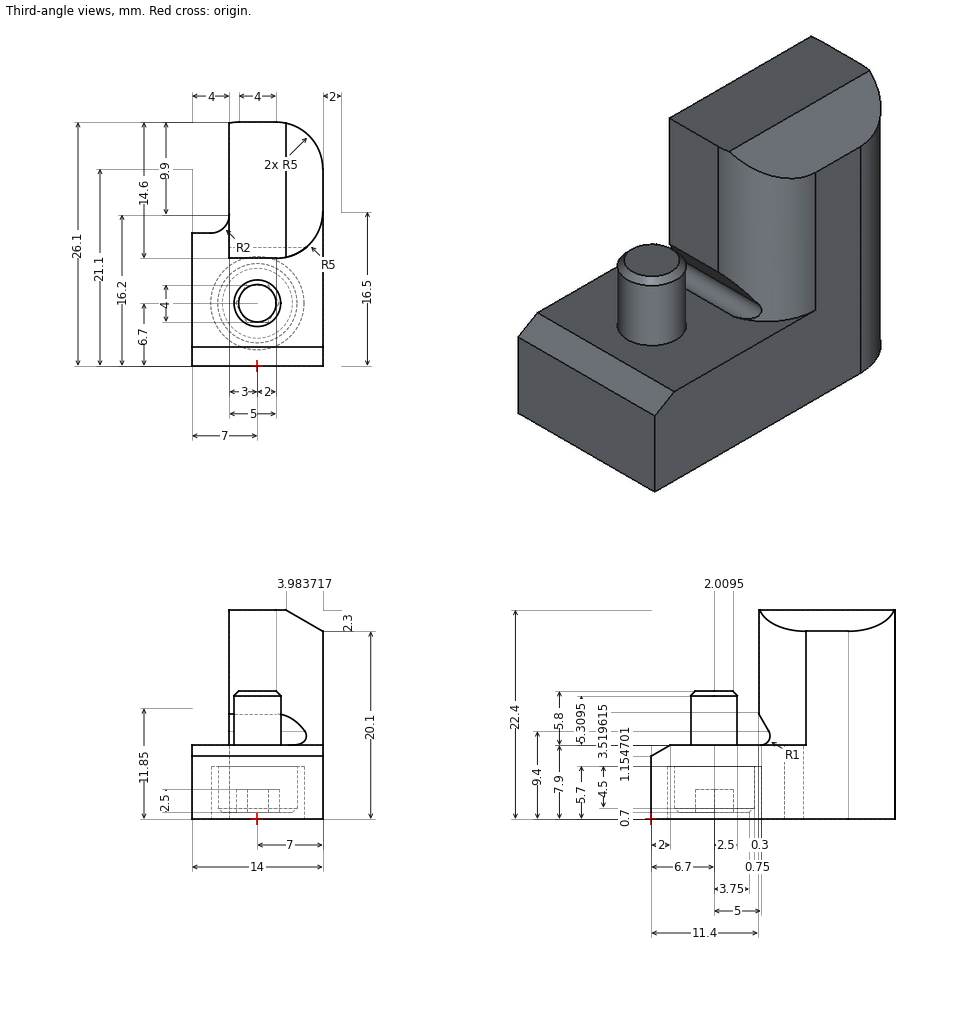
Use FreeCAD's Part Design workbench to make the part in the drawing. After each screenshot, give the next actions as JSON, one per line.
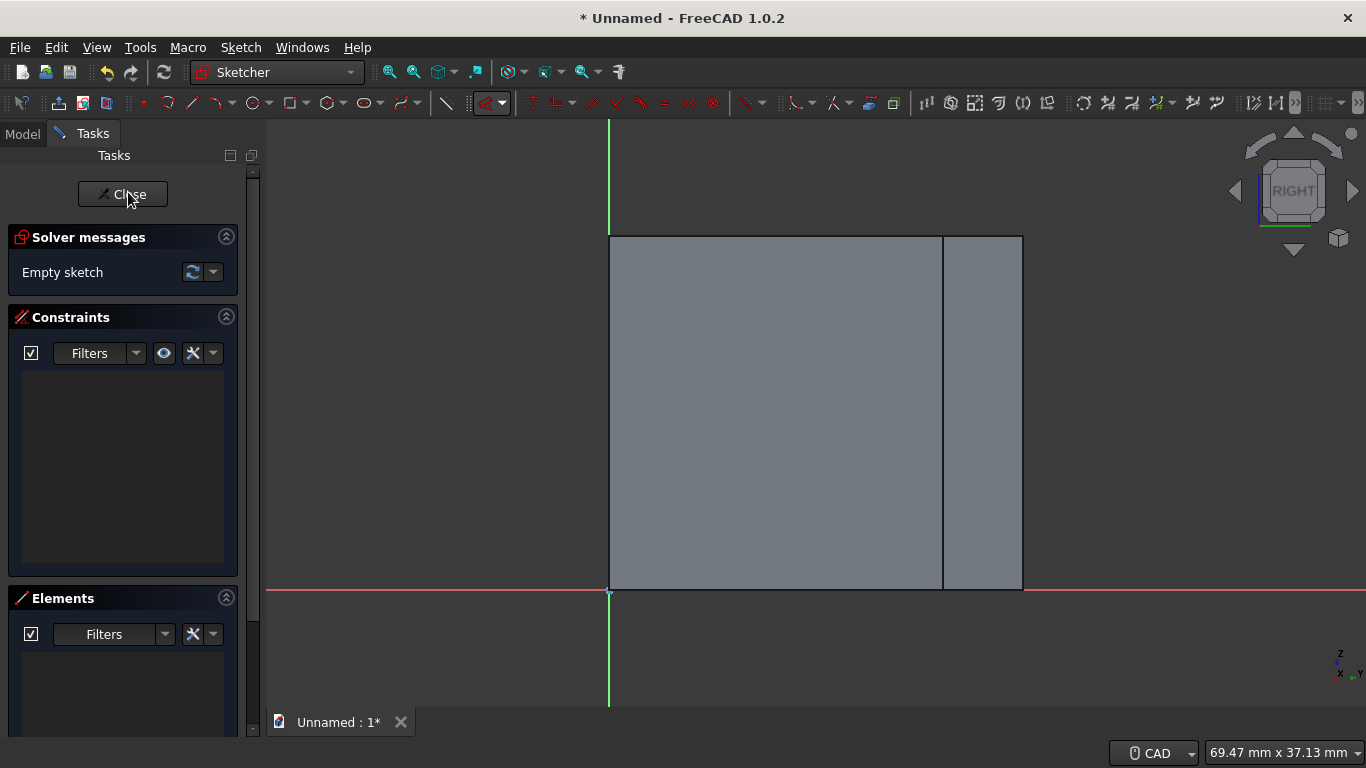
{"action": "left_click", "coordinate": [108, 104]}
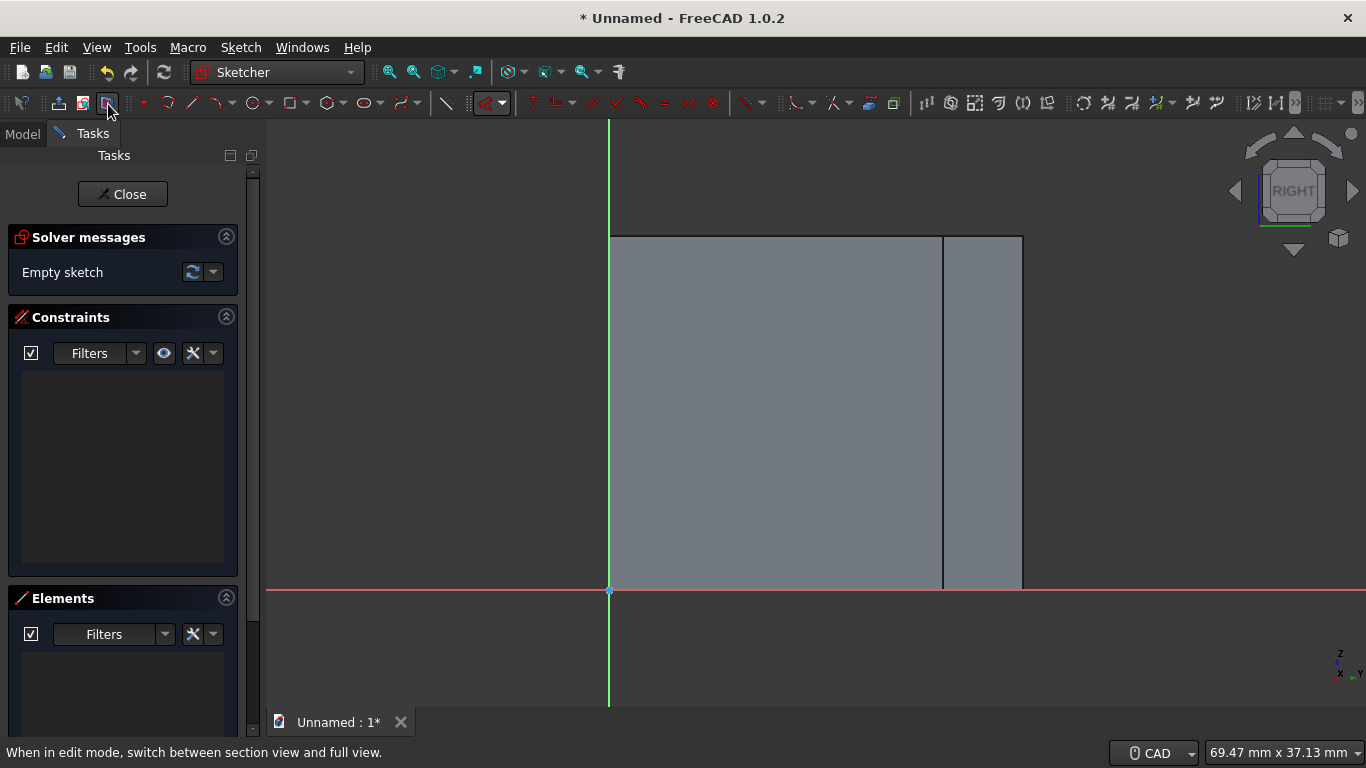
{"action": "scroll", "coordinate": [619, 478], "scroll_direction": "up", "scroll_amount": 15}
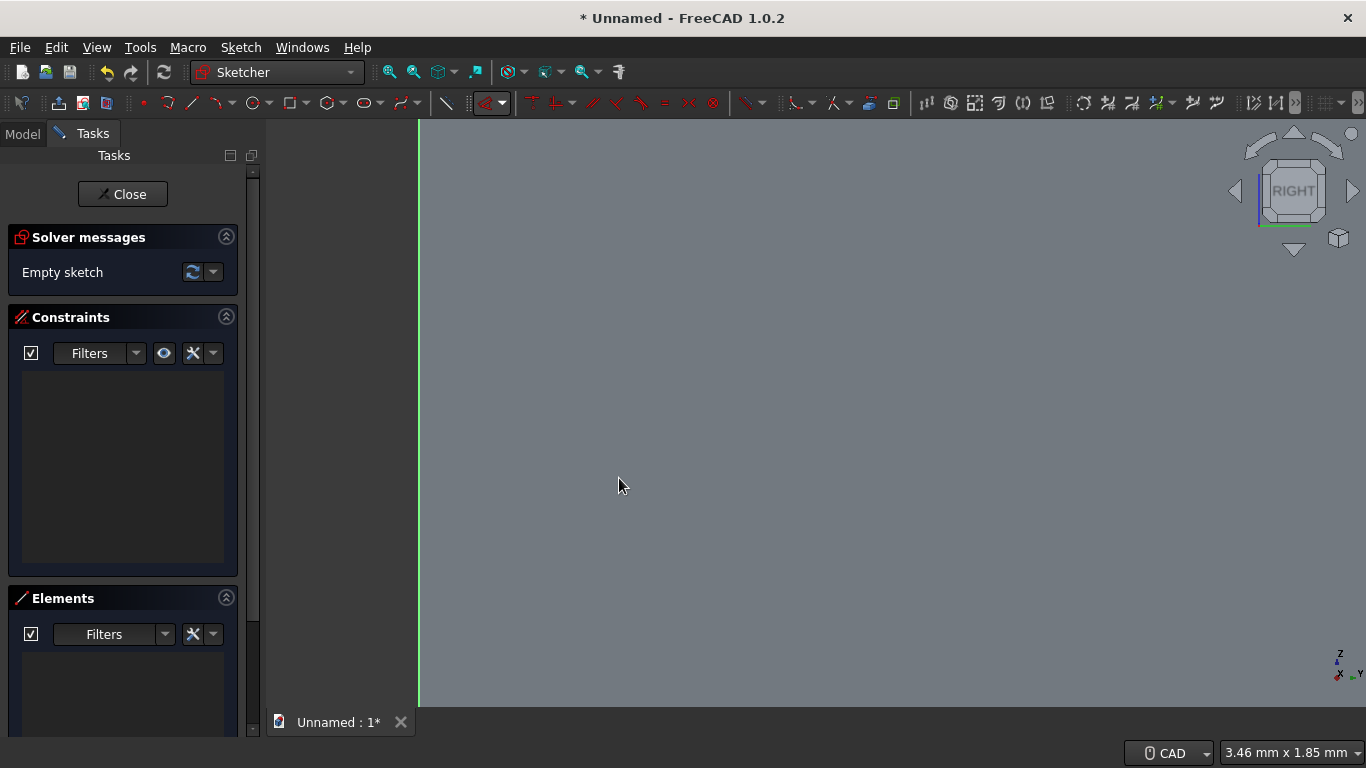
{"action": "left_click", "coordinate": [168, 104]}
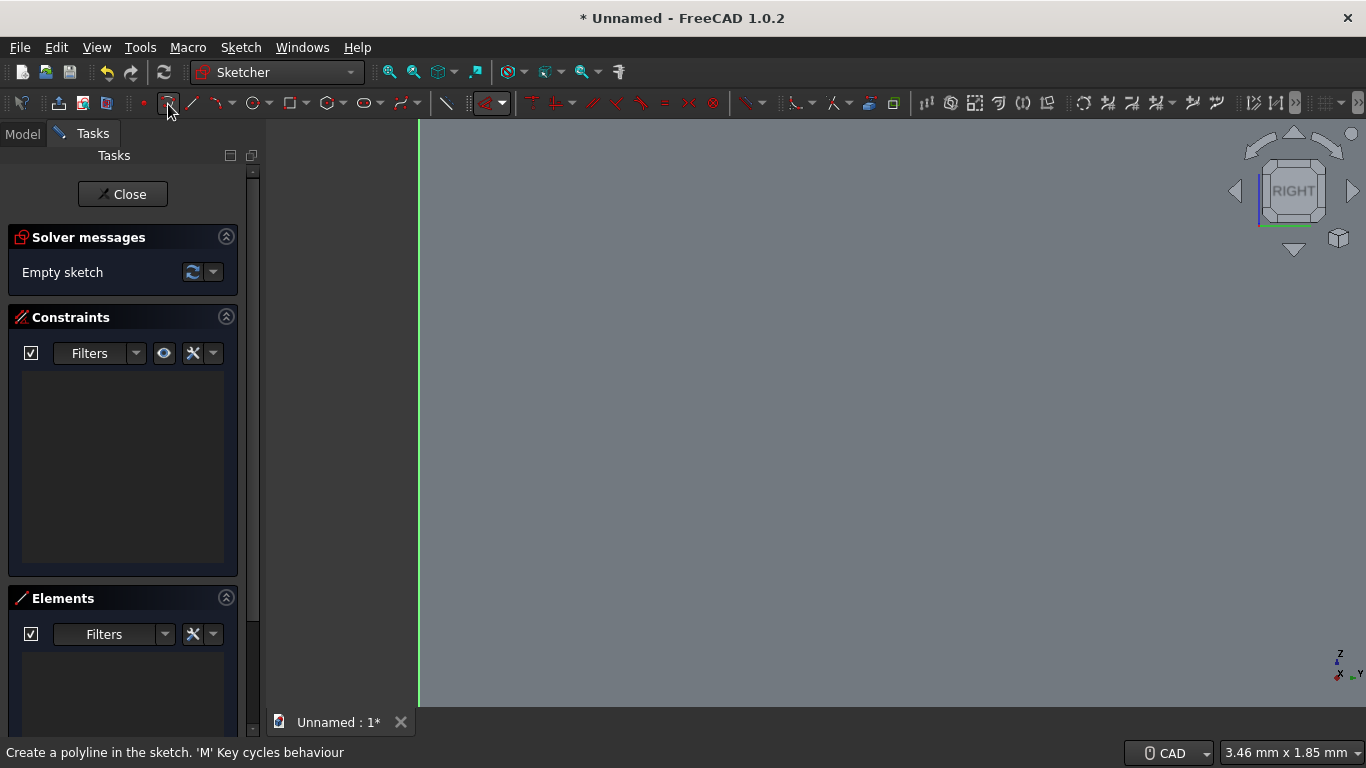
{"action": "left_click", "coordinate": [419, 578]}
{"action": "left_click", "coordinate": [1055, 210]}
{"action": "left_click", "coordinate": [428, 210]}
{"action": "left_click", "coordinate": [419, 579]}
{"action": "key", "text": "Escape"}
{"action": "key", "text": "Escape"}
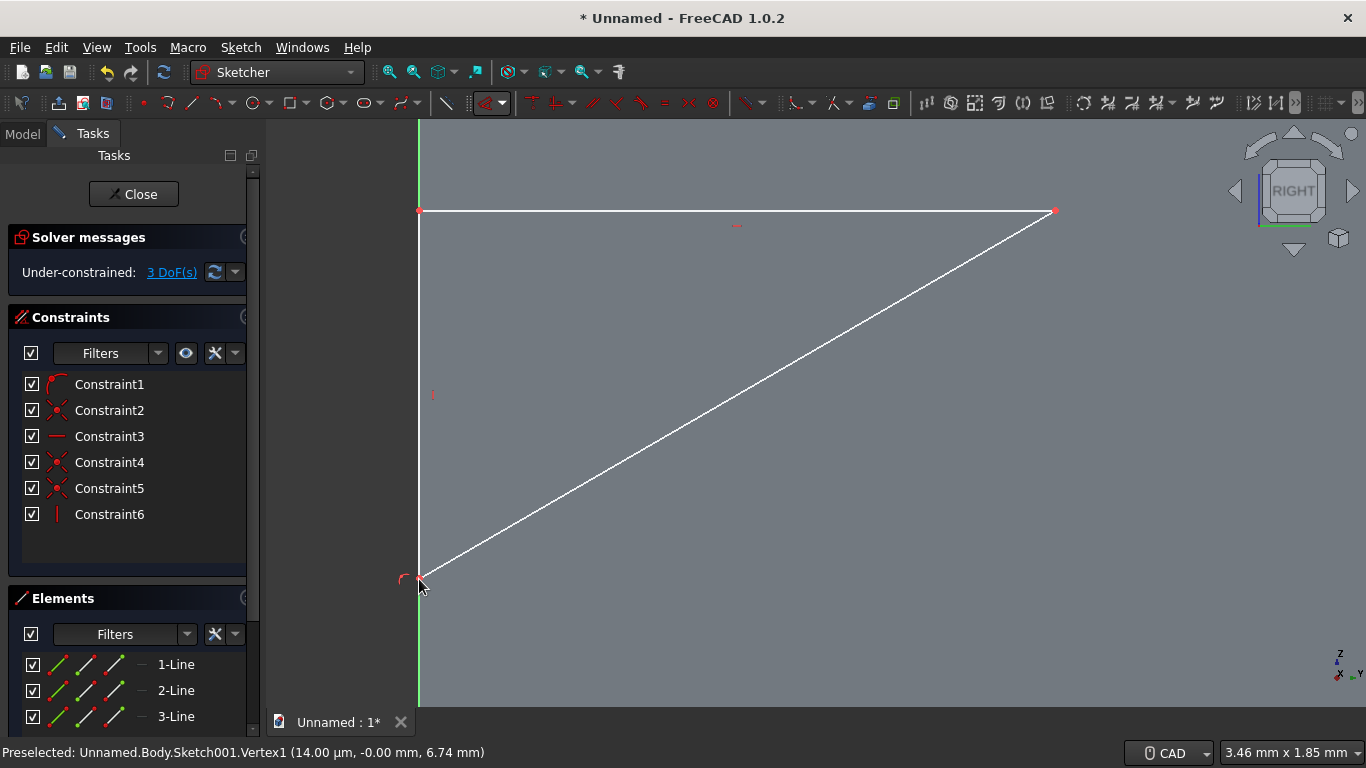
{"action": "left_click", "coordinate": [864, 211]}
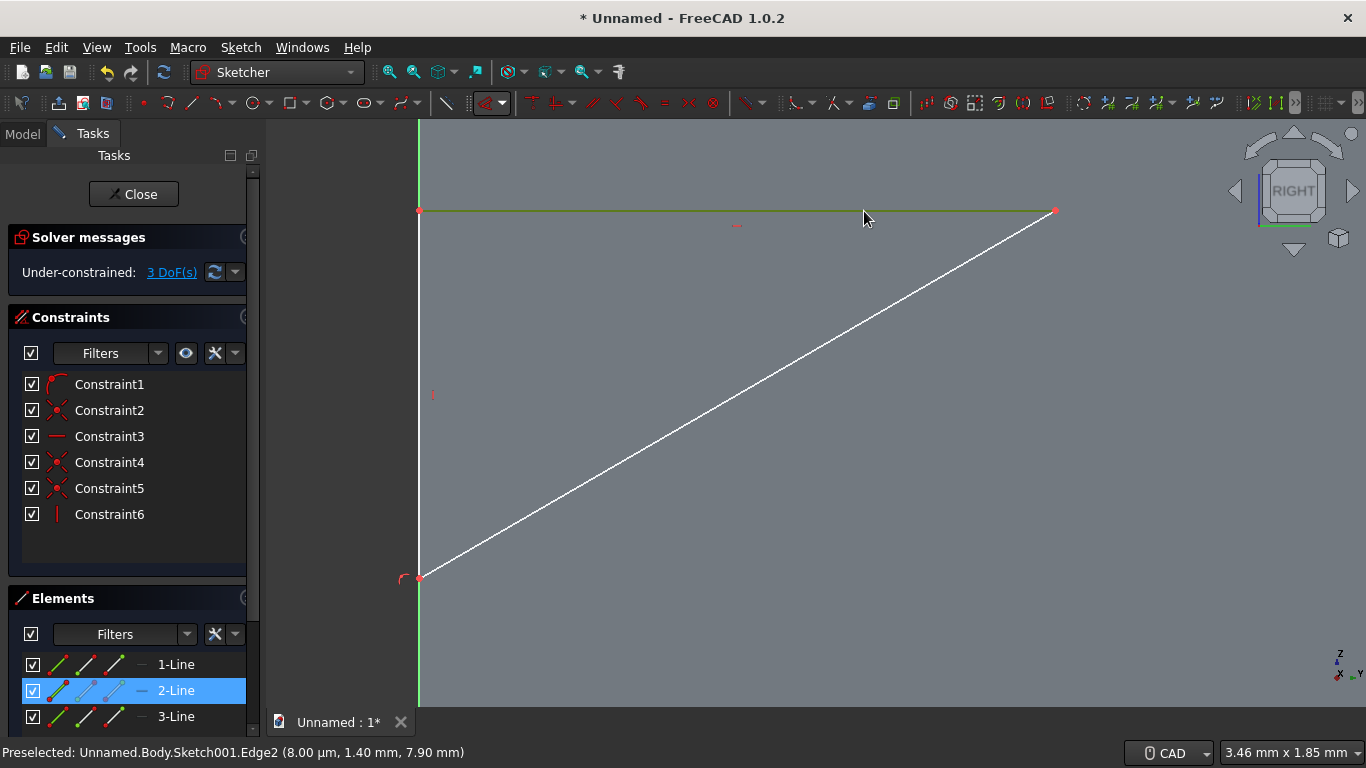
{"action": "left_click", "coordinate": [504, 104]}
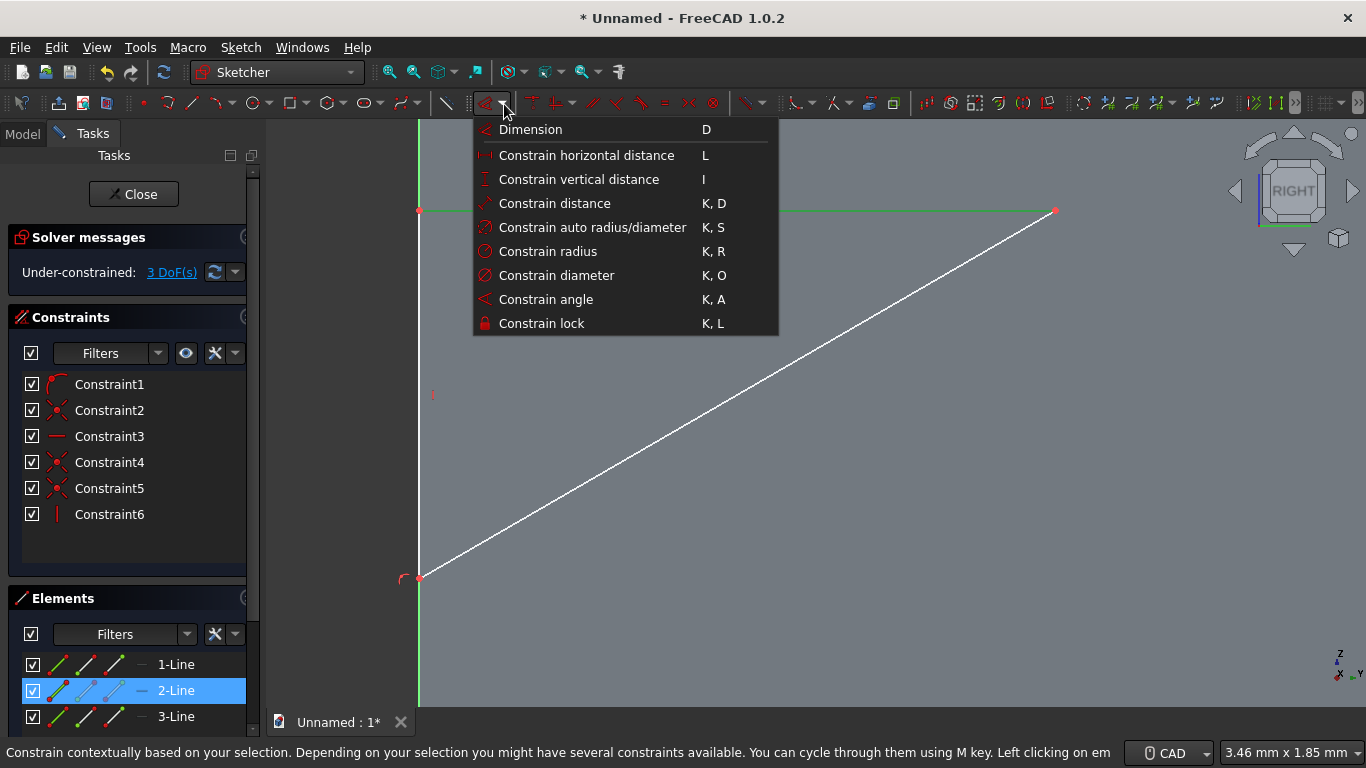
{"action": "left_click", "coordinate": [626, 155]}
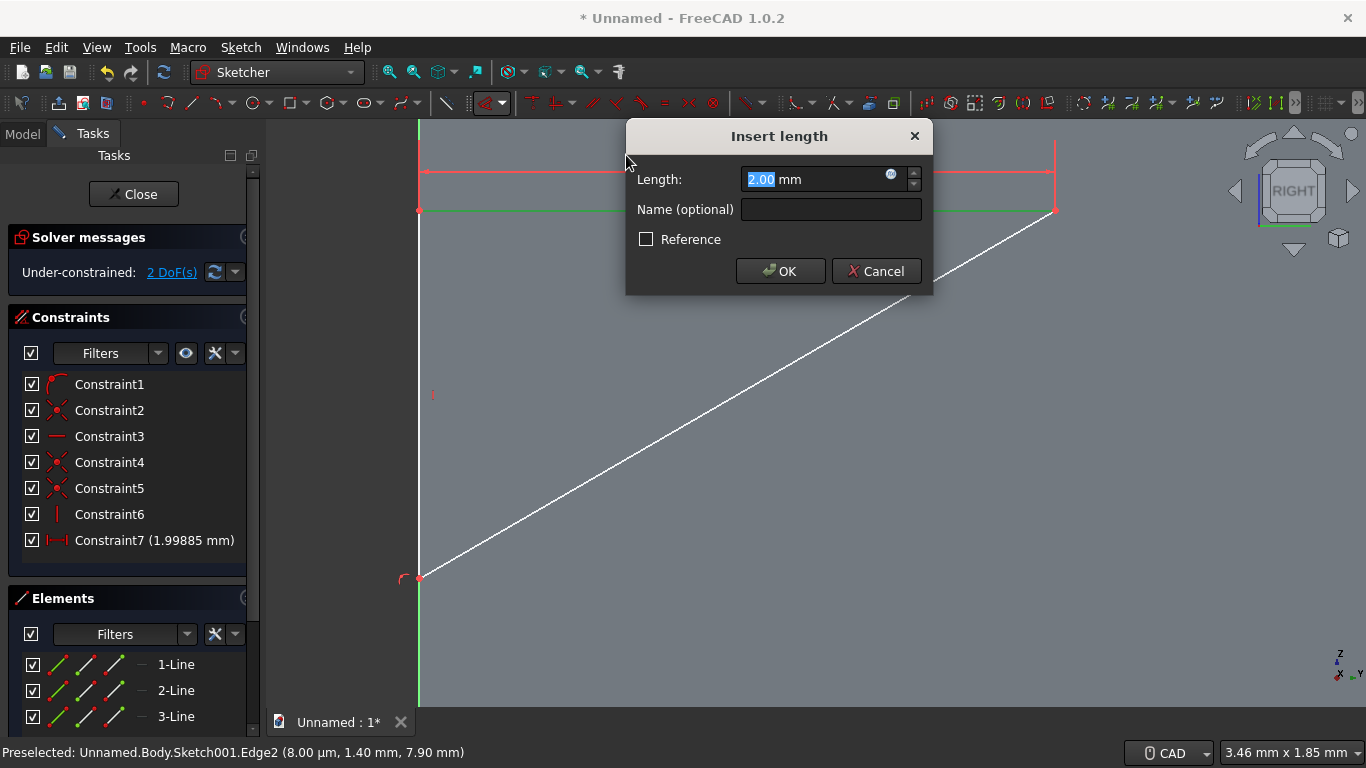
{"action": "type", "text": "2"}
{"action": "key", "text": "Return"}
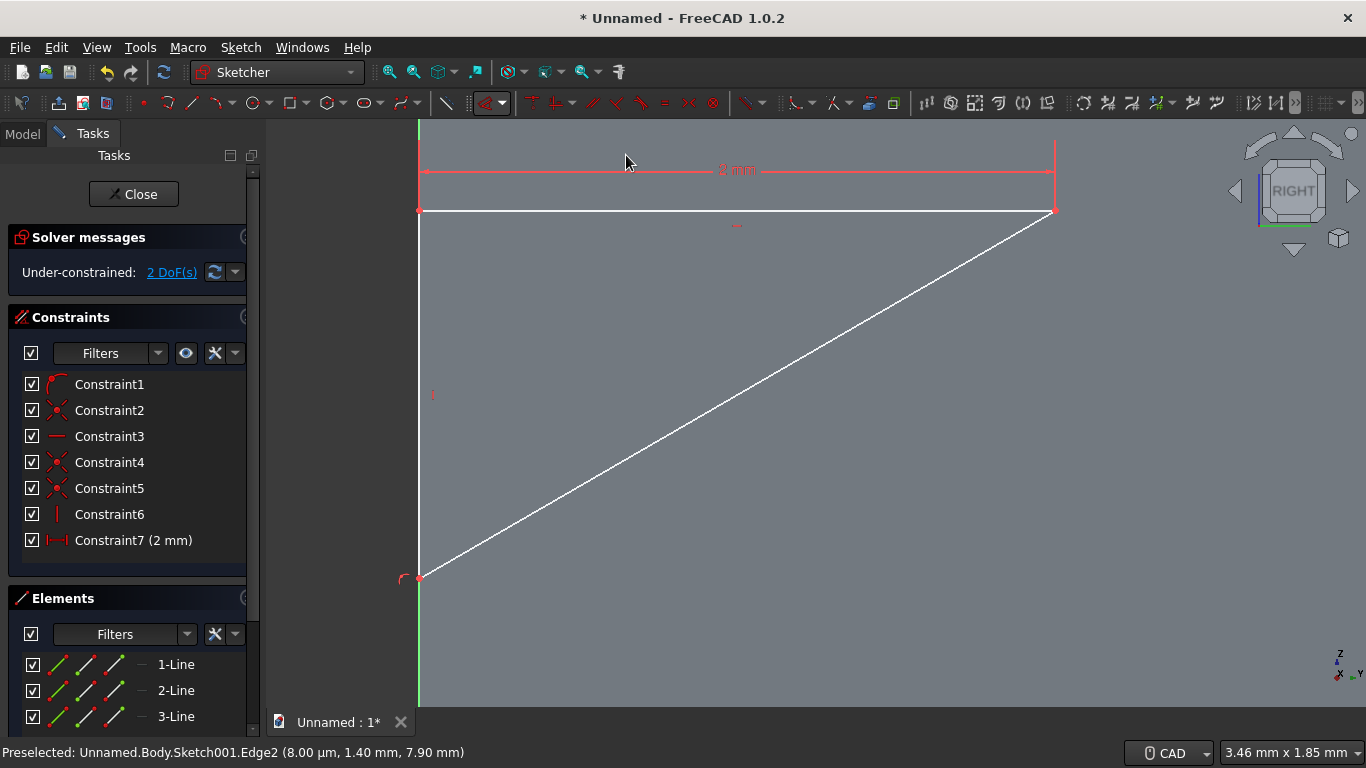
{"action": "left_click", "coordinate": [1055, 211]}